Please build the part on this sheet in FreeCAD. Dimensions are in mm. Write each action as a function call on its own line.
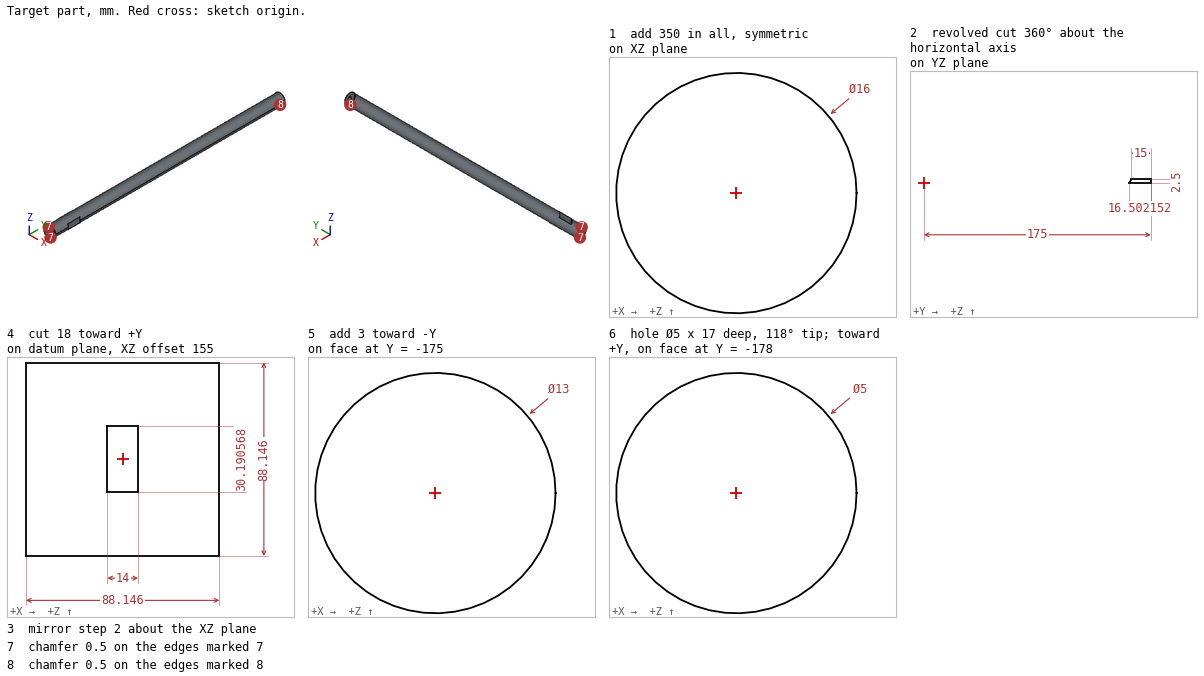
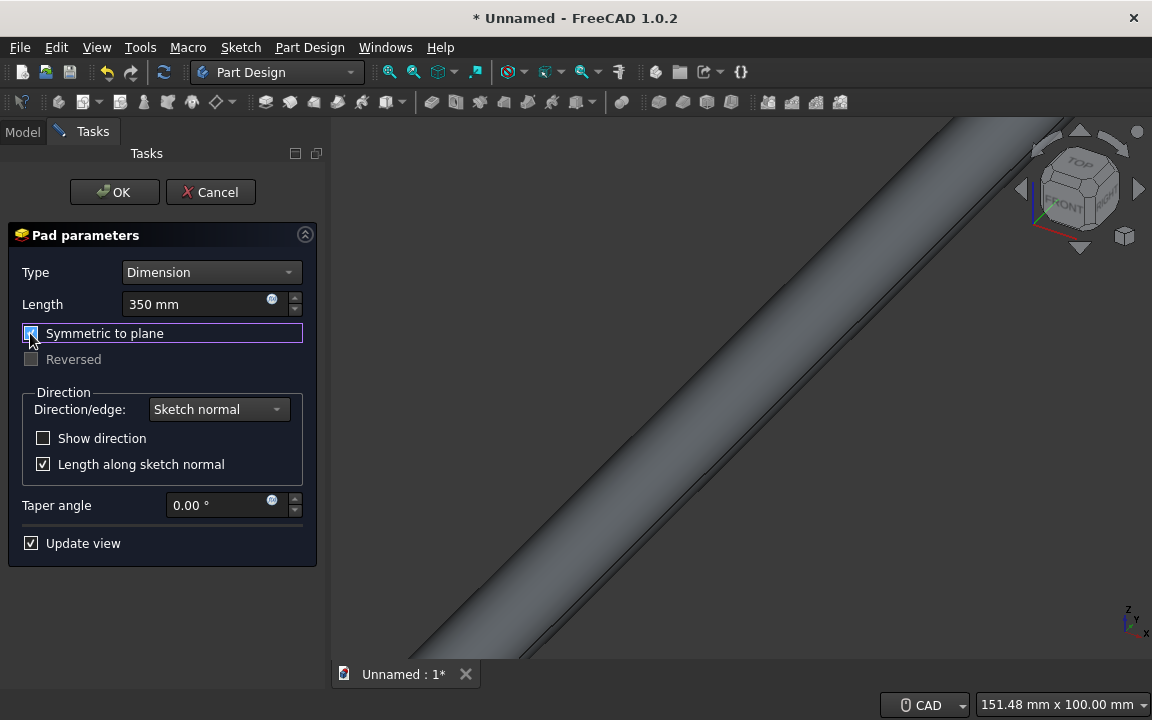
click(115, 192)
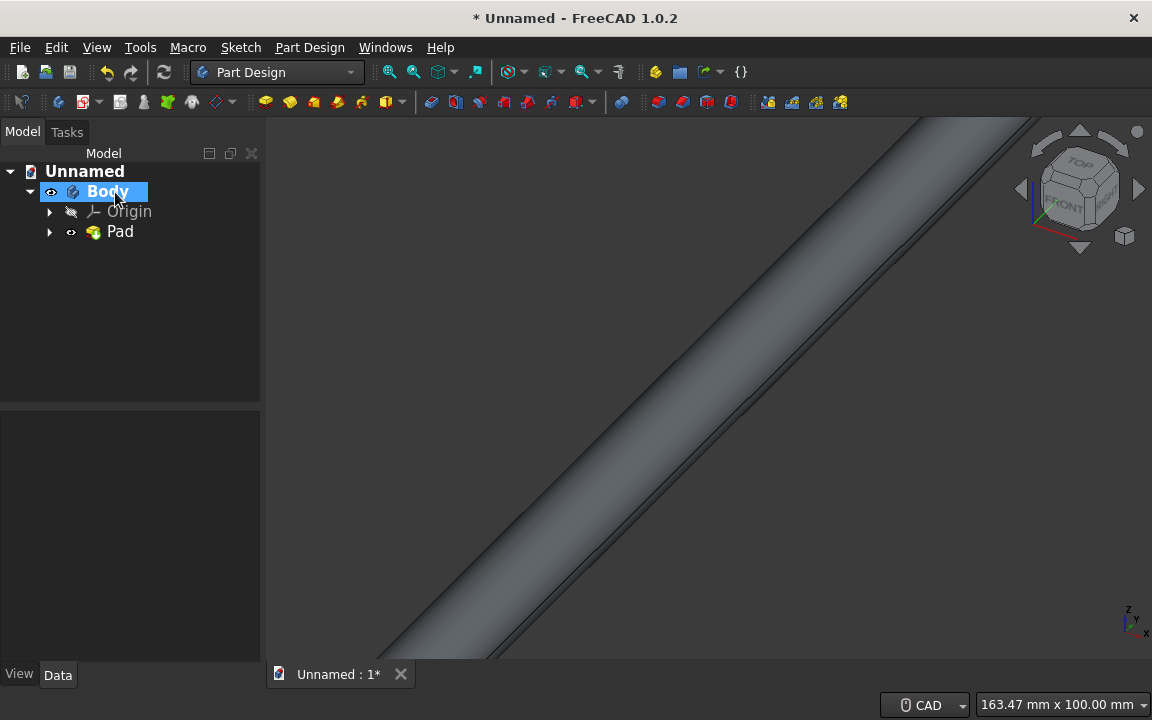
click(390, 72)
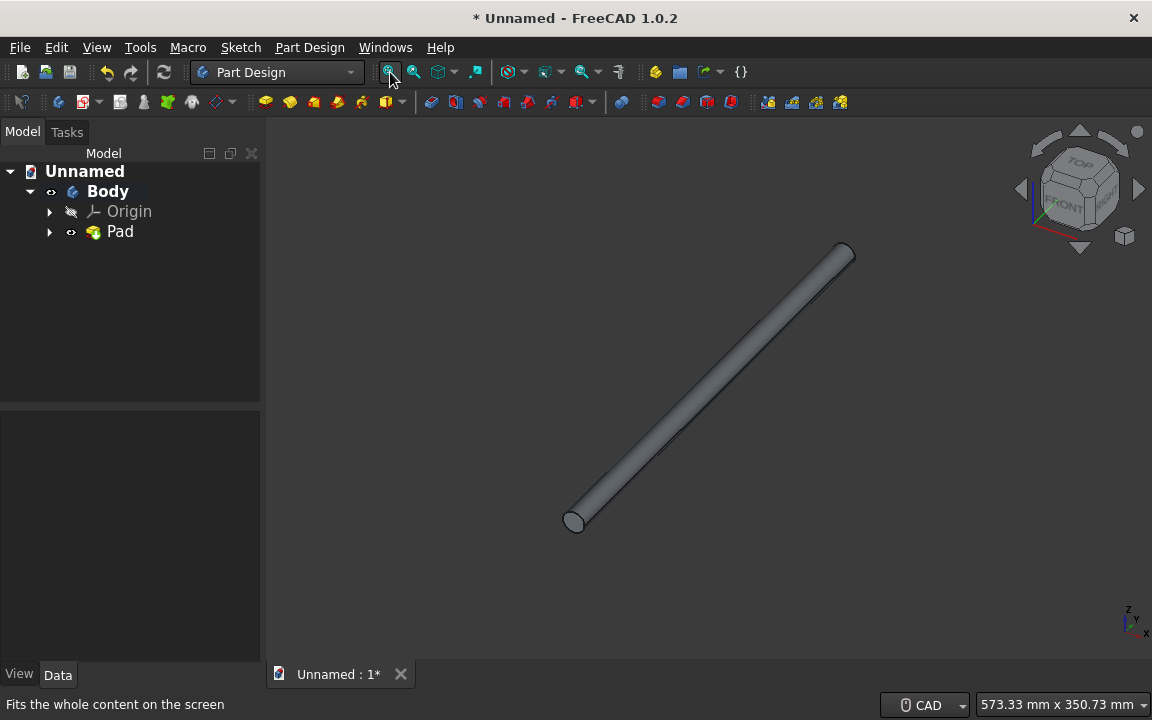
click(84, 102)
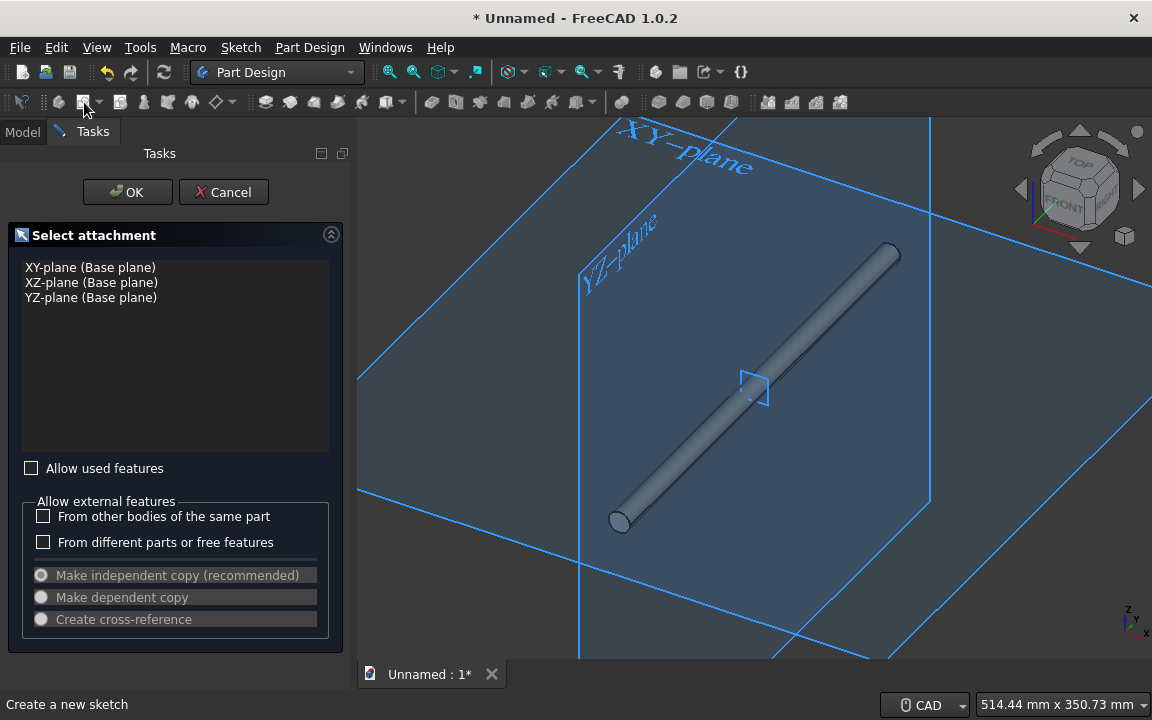
click(82, 298)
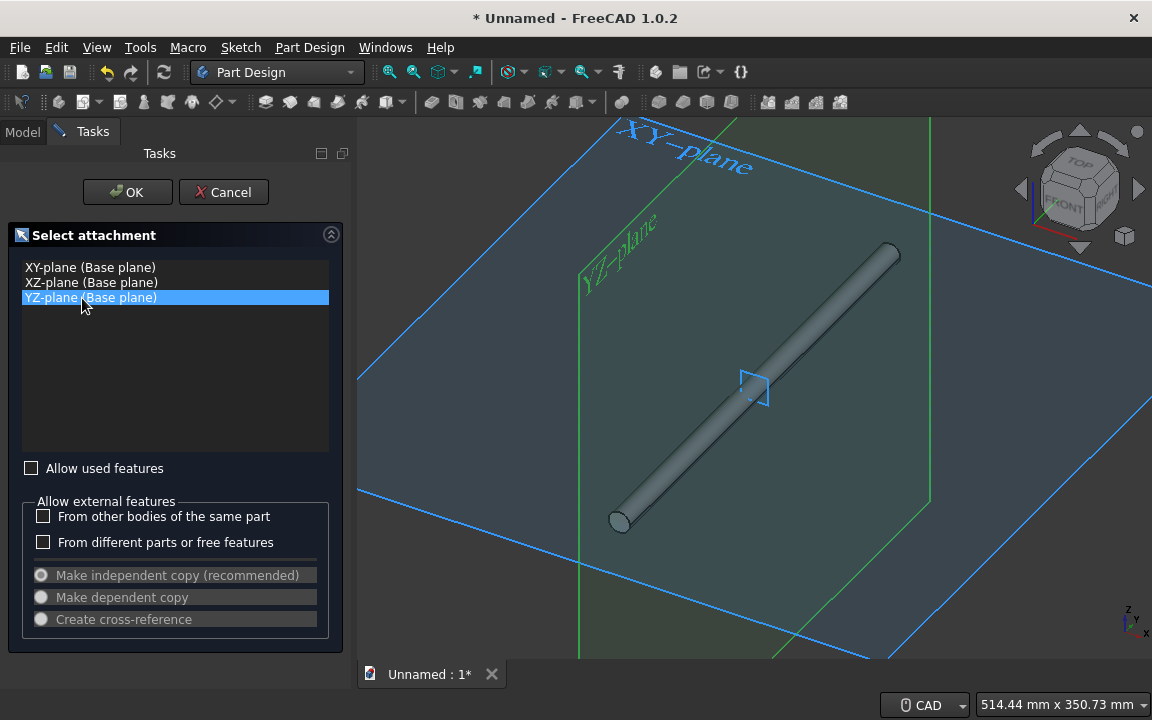
click(128, 192)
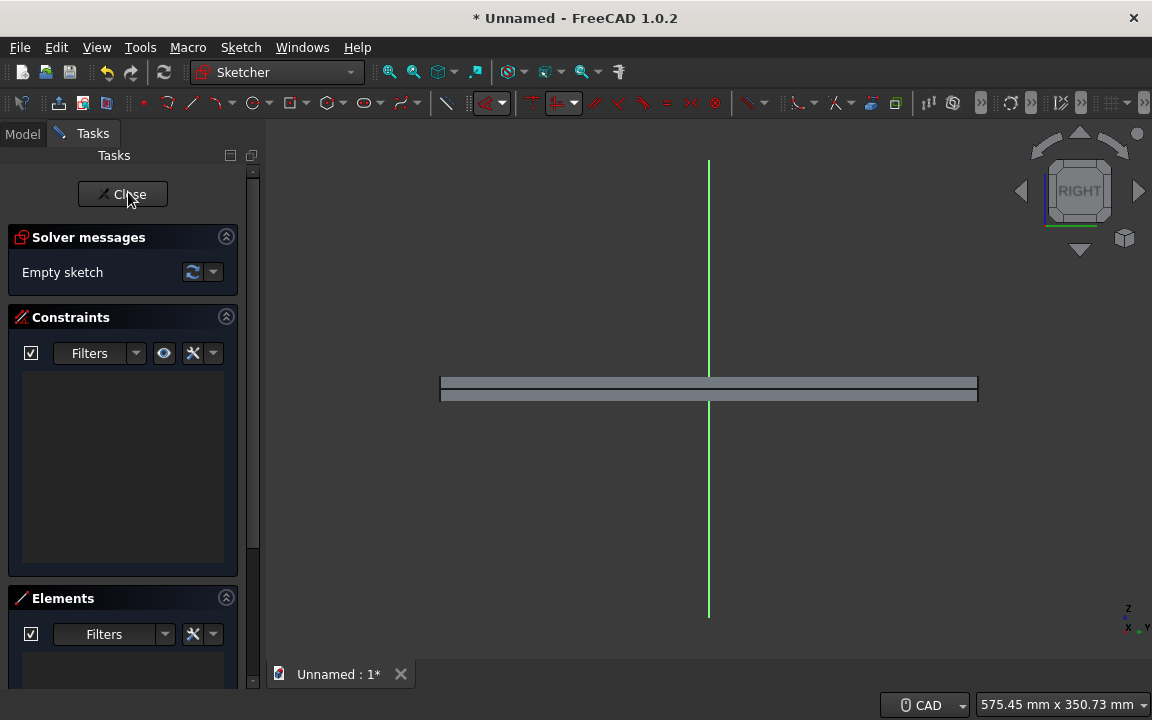
click(108, 104)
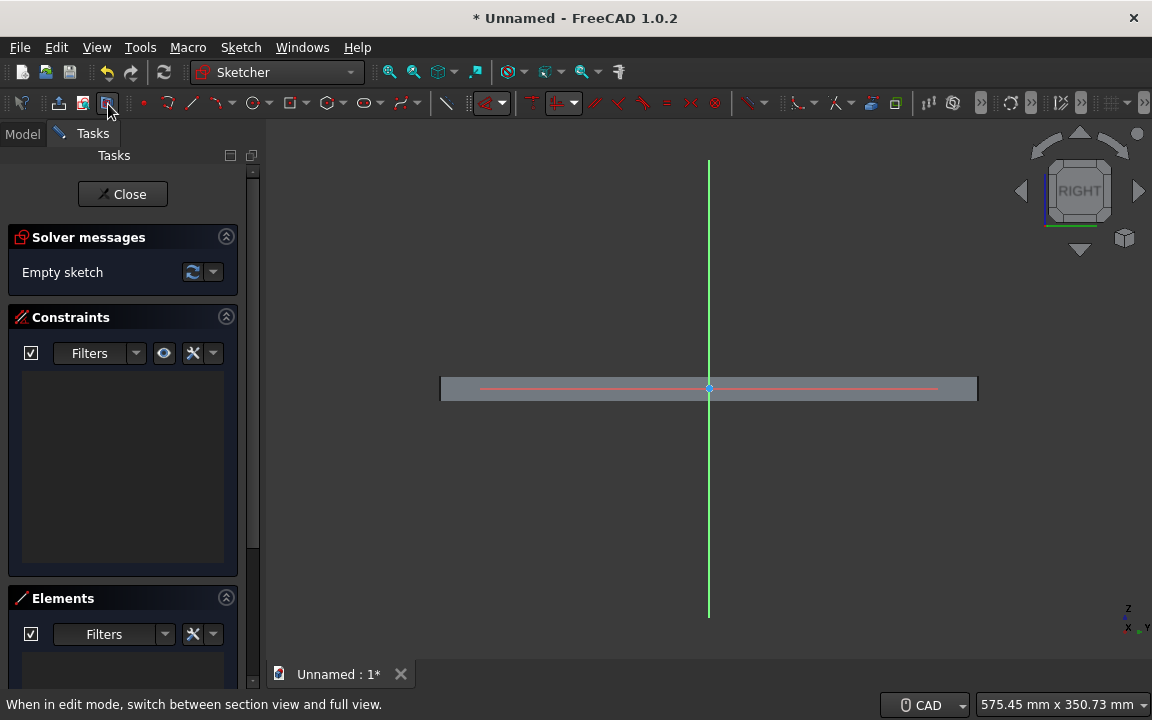
scroll(983, 387, up, 15)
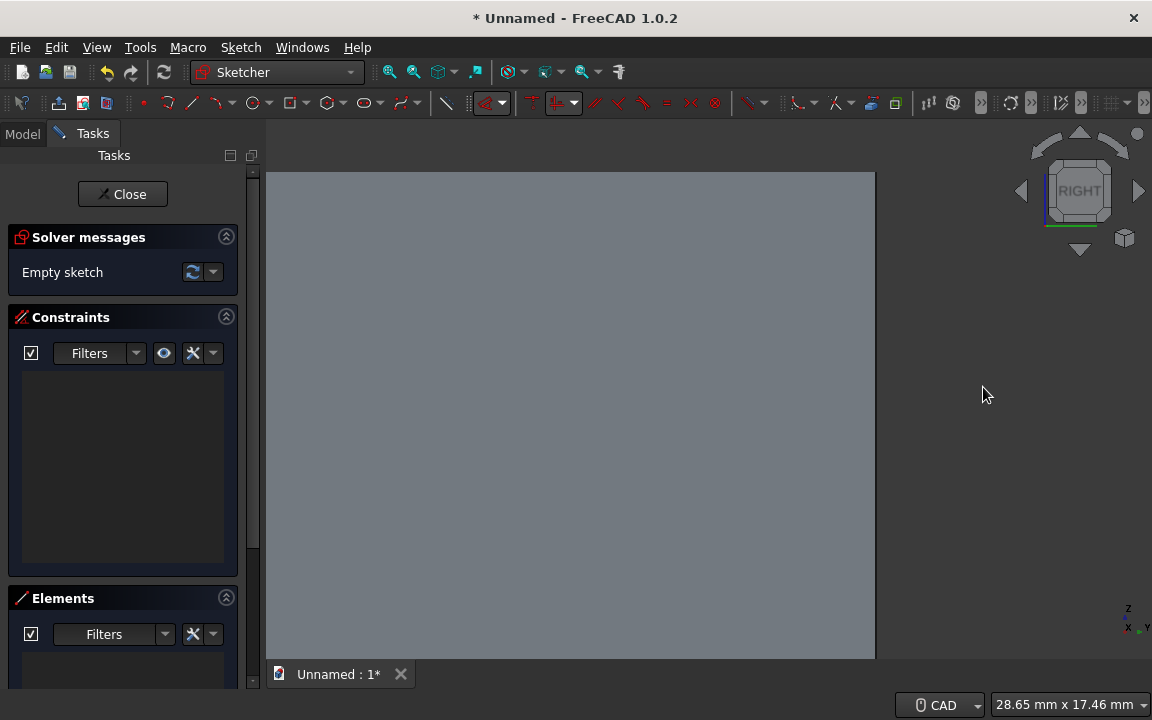
click(168, 104)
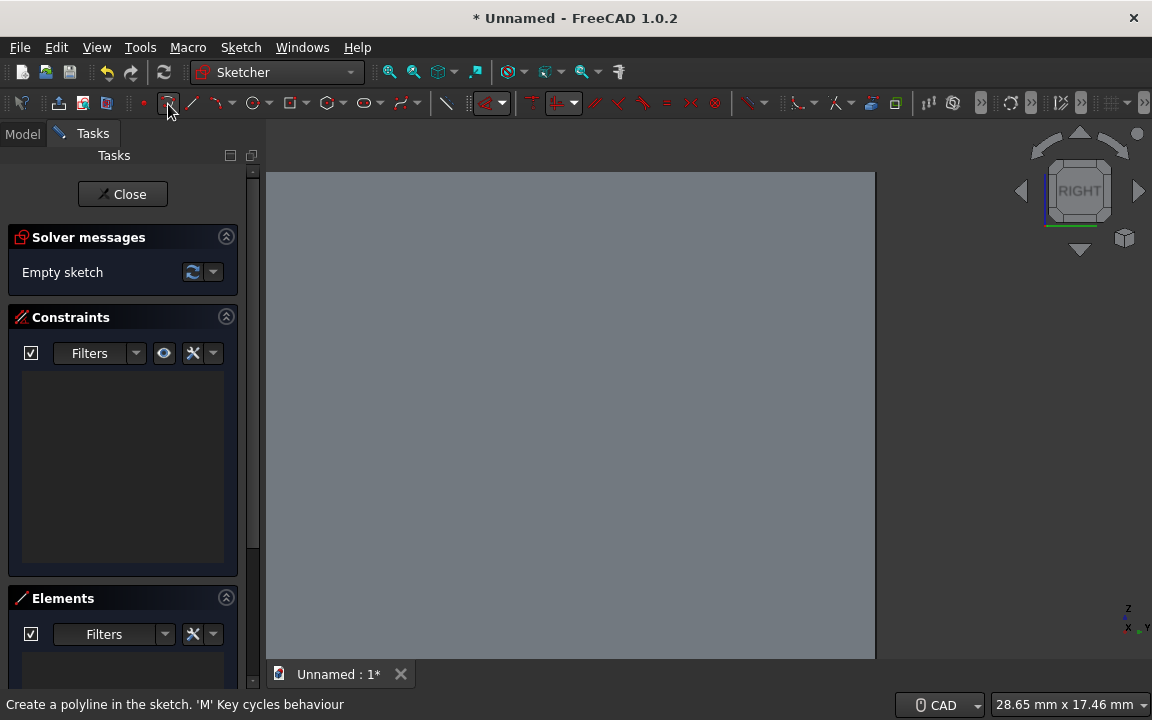
click(366, 418)
click(876, 409)
click(876, 340)
click(412, 340)
click(366, 419)
key(Escape)
key(Escape)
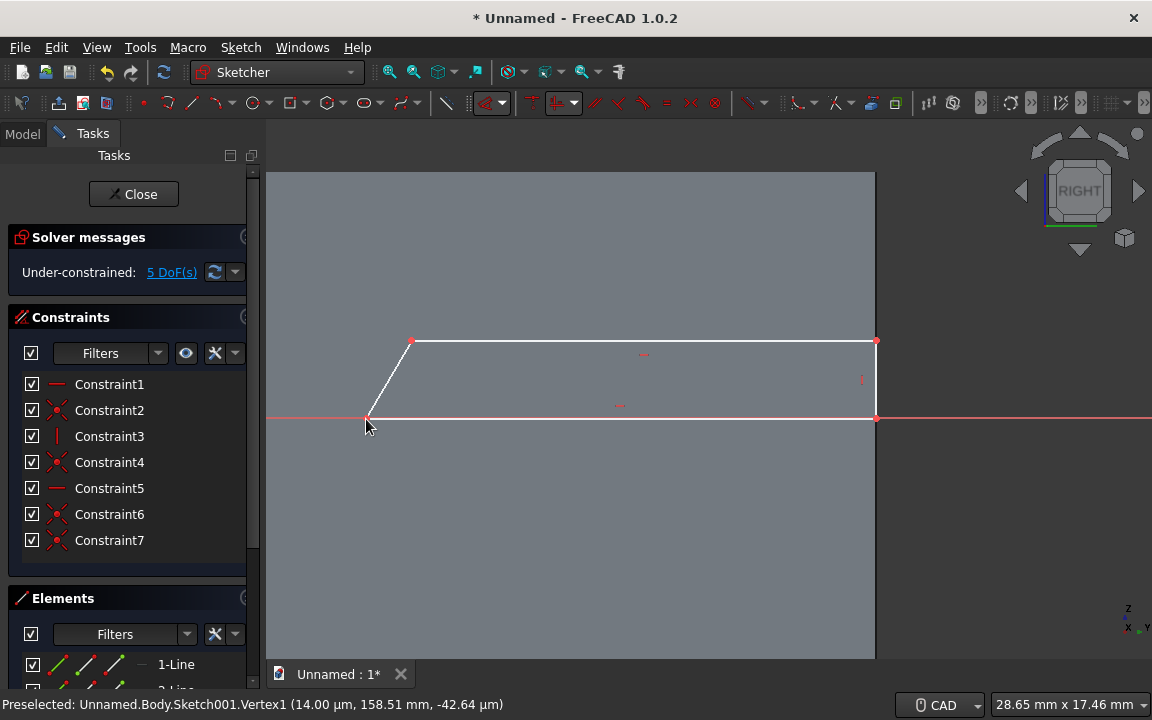
click(366, 419)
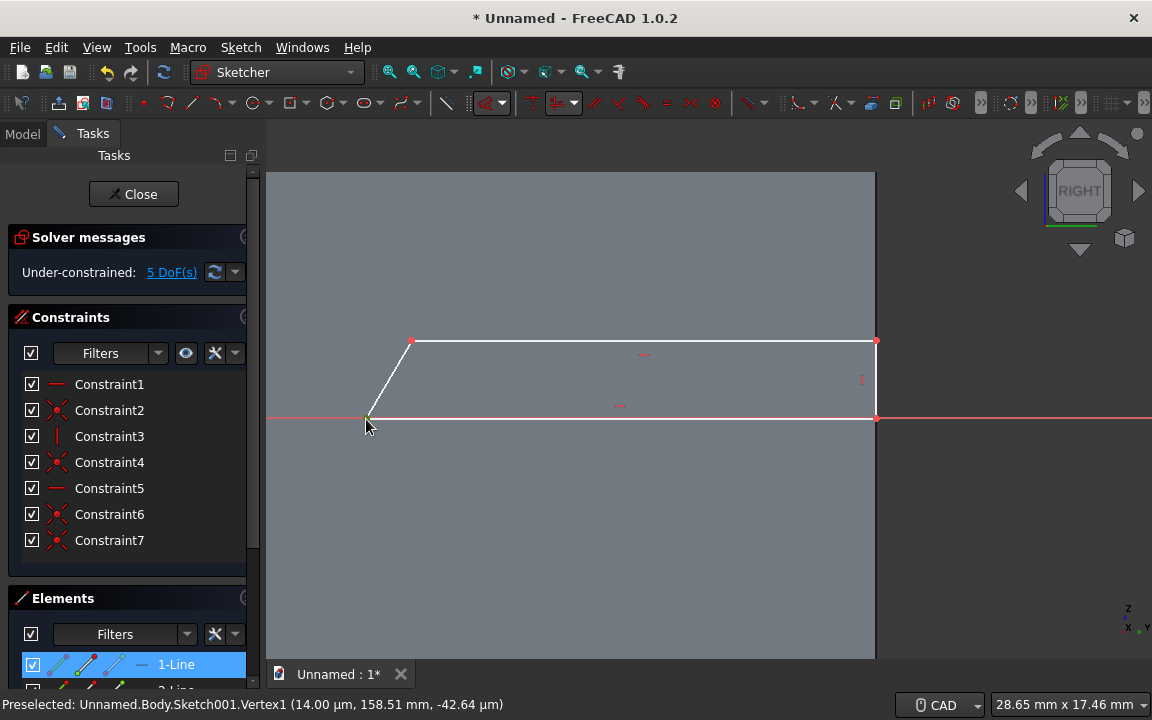
click(938, 418)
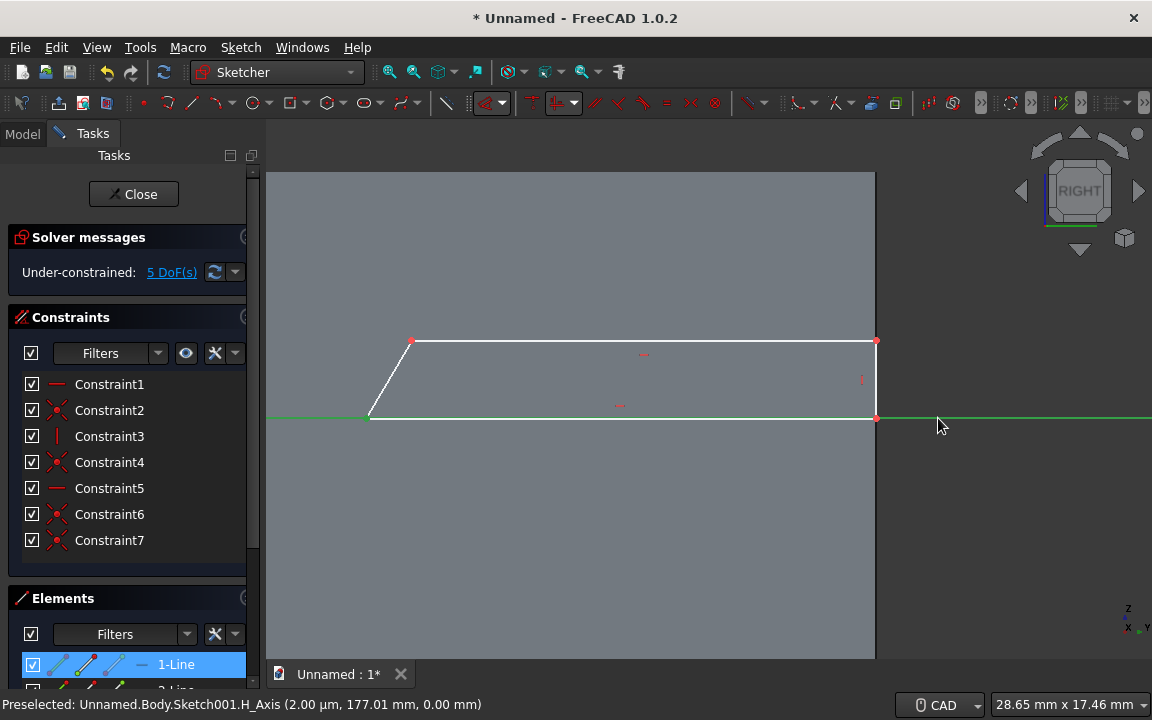
key(c)